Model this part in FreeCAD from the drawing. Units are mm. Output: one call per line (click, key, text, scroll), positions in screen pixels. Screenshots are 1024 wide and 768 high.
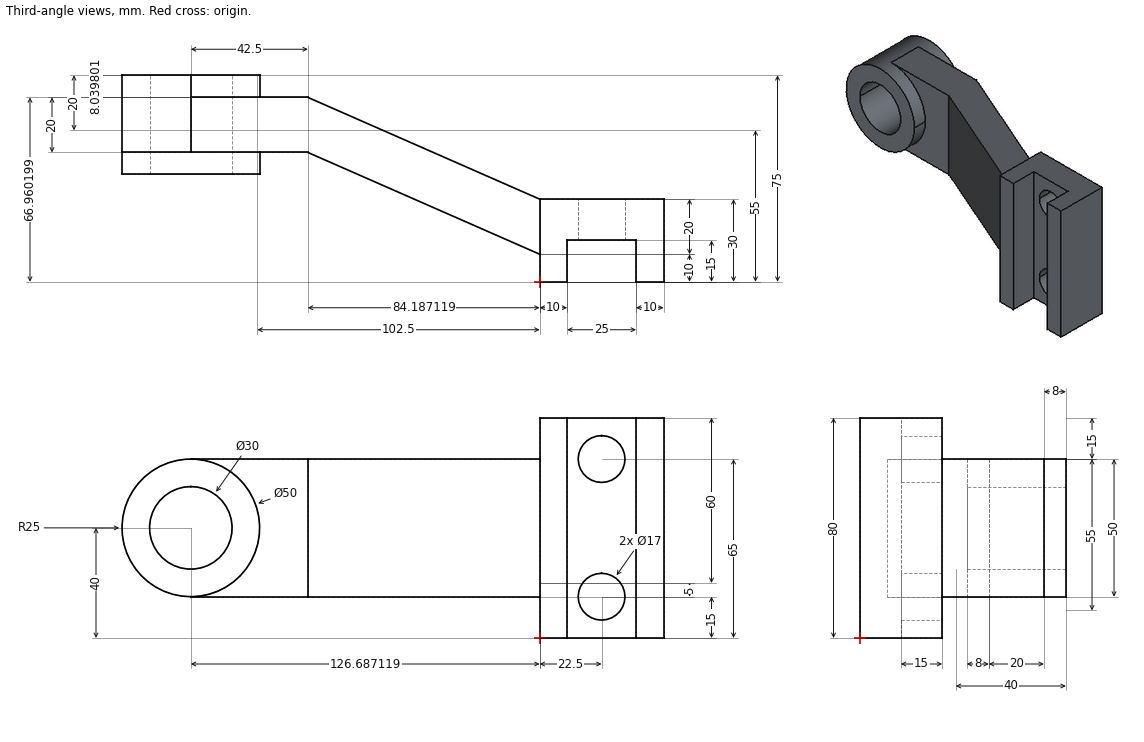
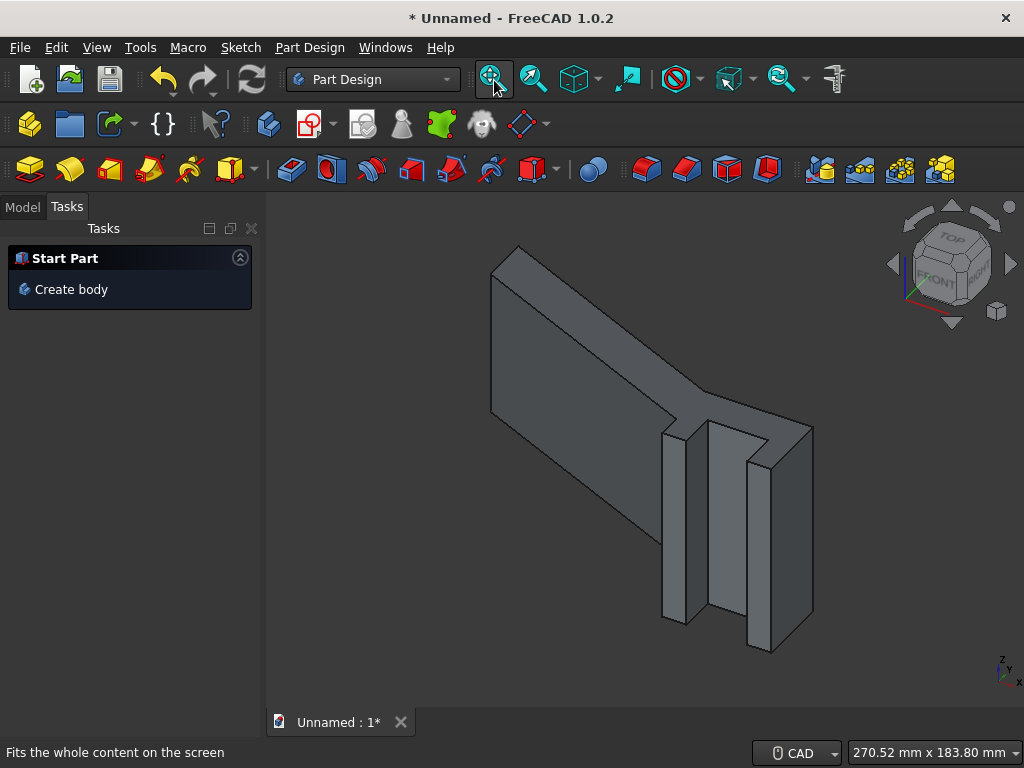
click(522, 276)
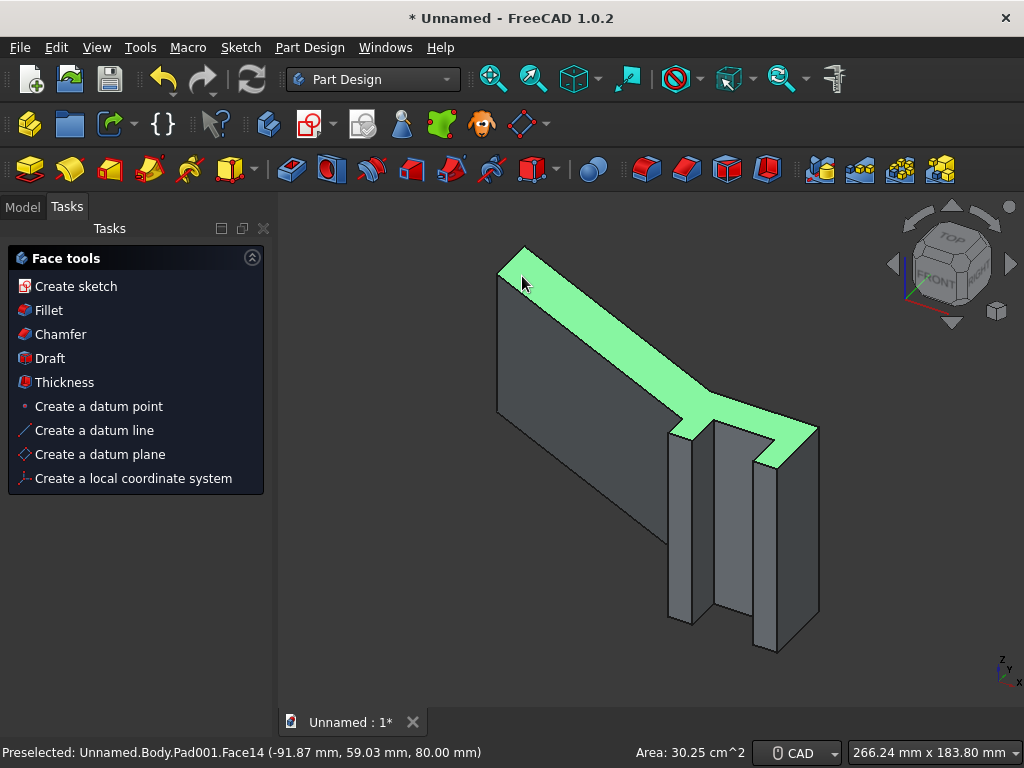
click(310, 124)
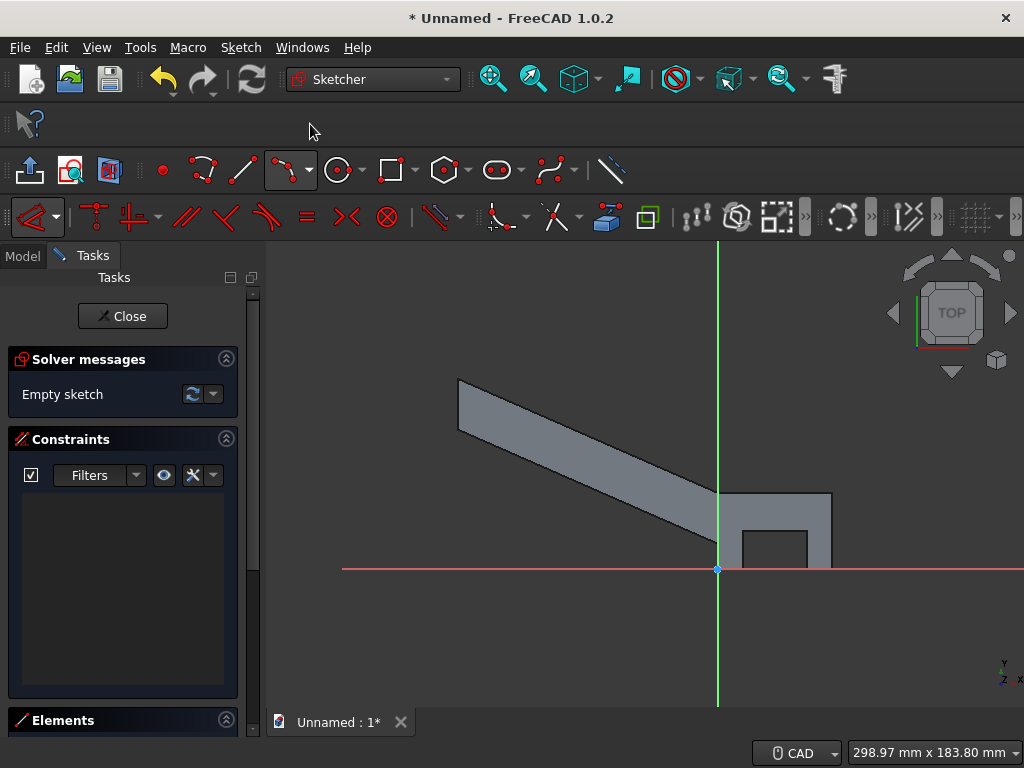
scroll(611, 474, up, 2)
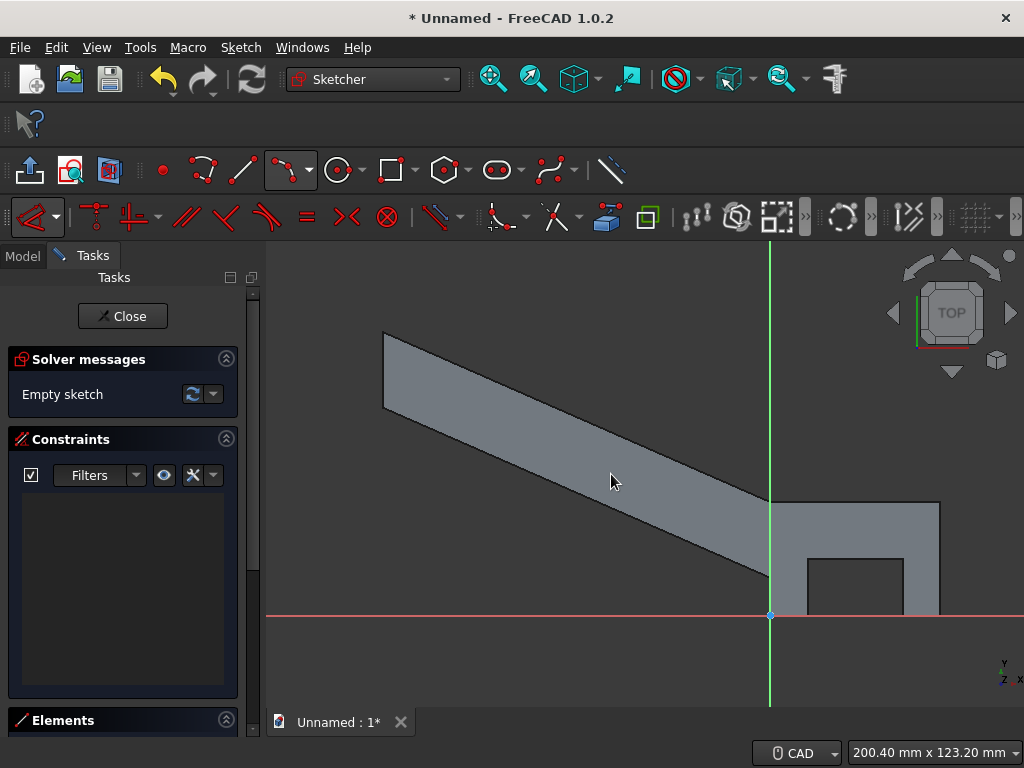
click(204, 170)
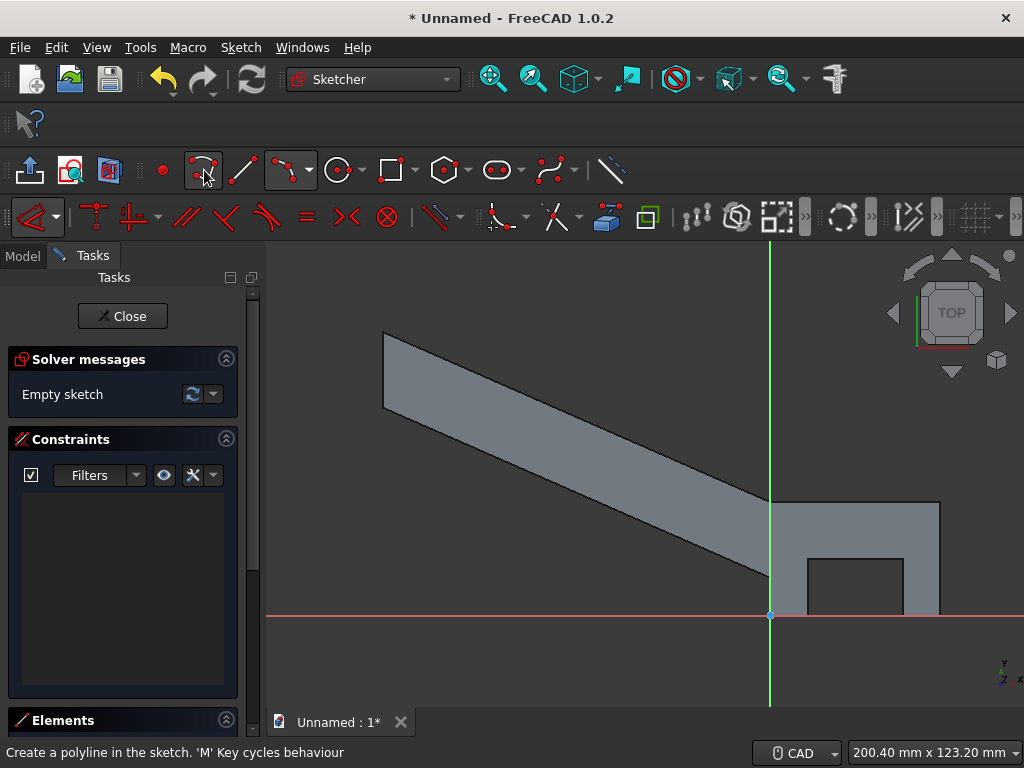
click(770, 578)
click(761, 502)
click(383, 332)
click(383, 408)
click(770, 579)
key(Escape)
key(Escape)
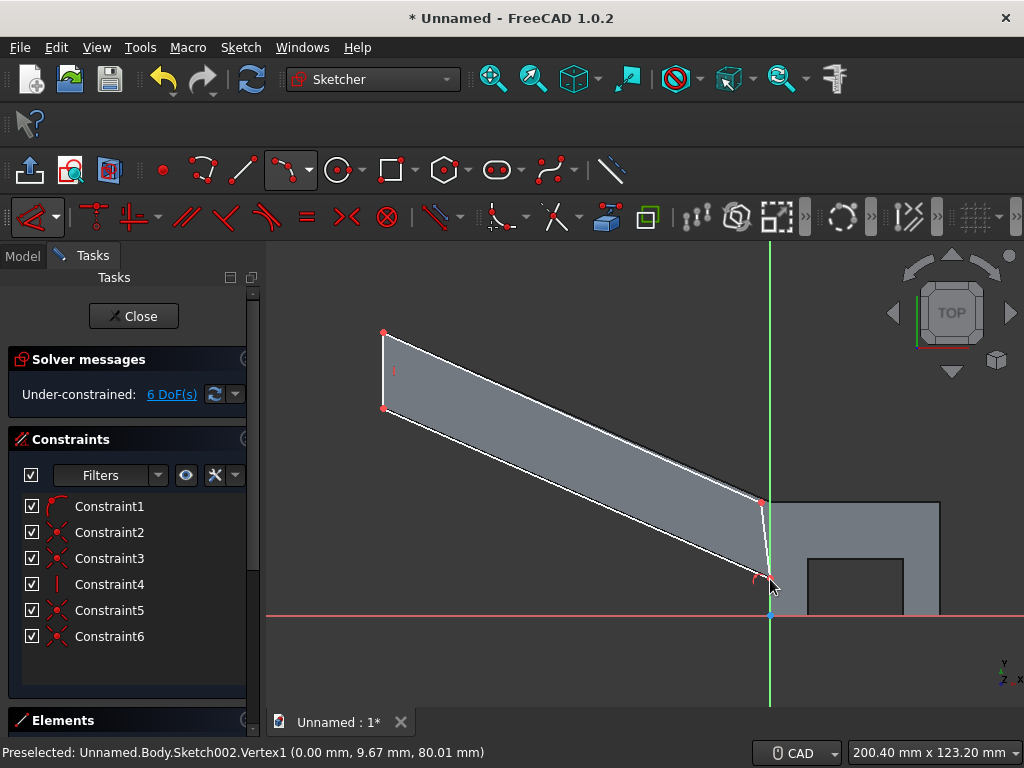
click(767, 556)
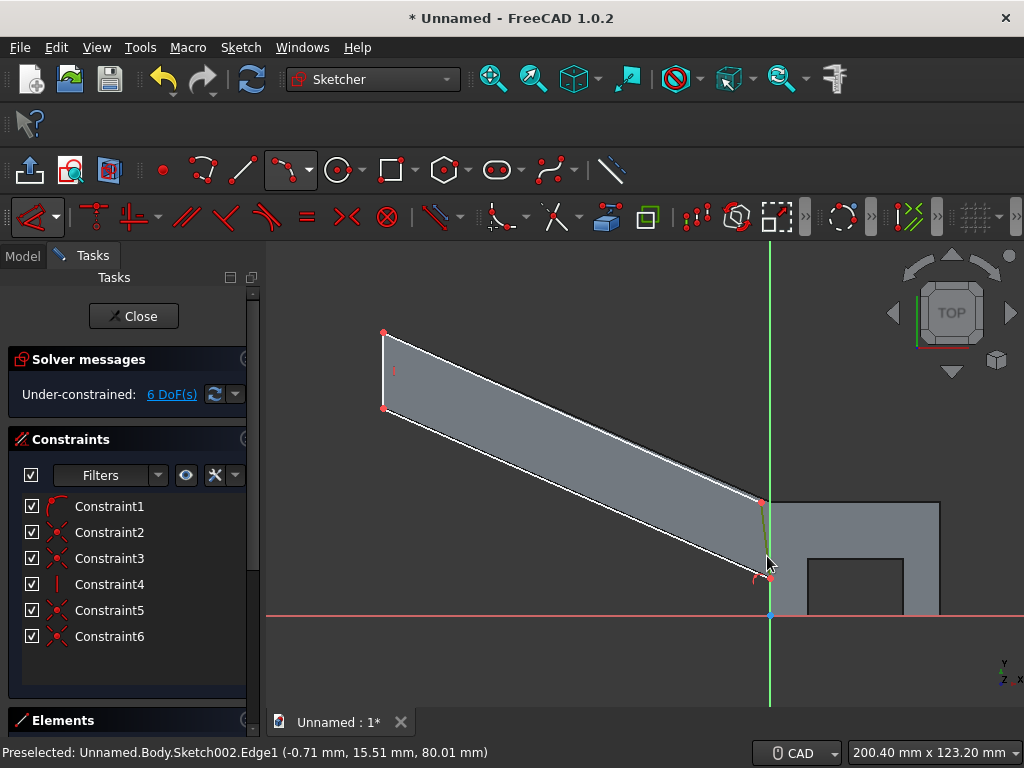
key(v)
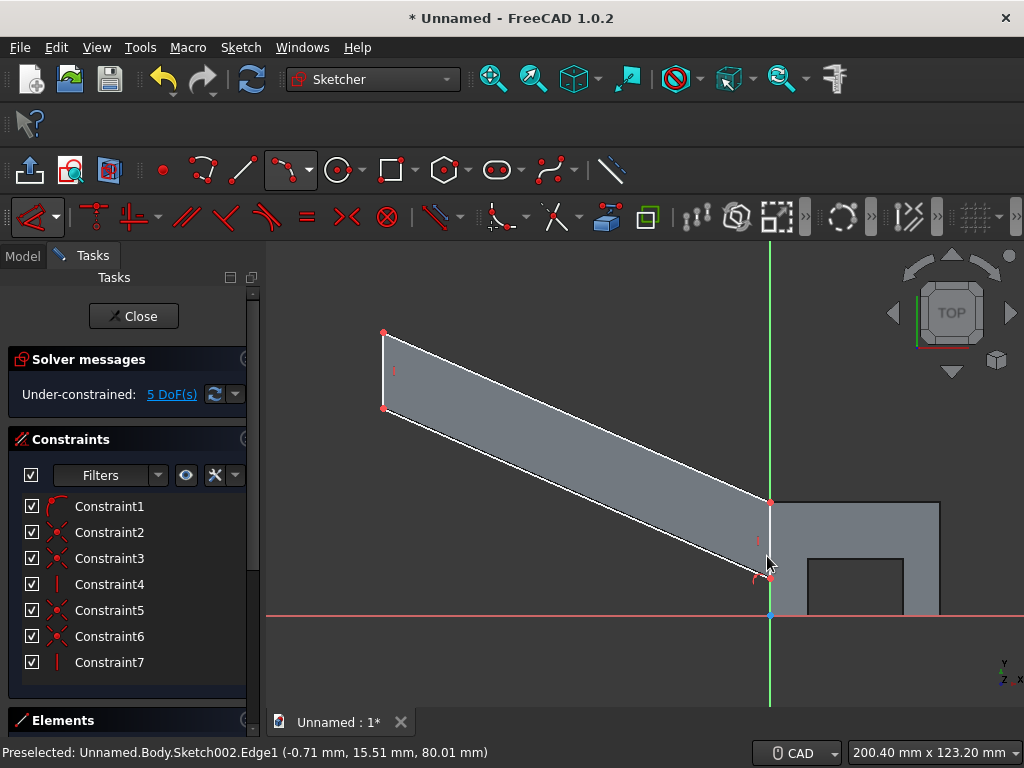
click(770, 556)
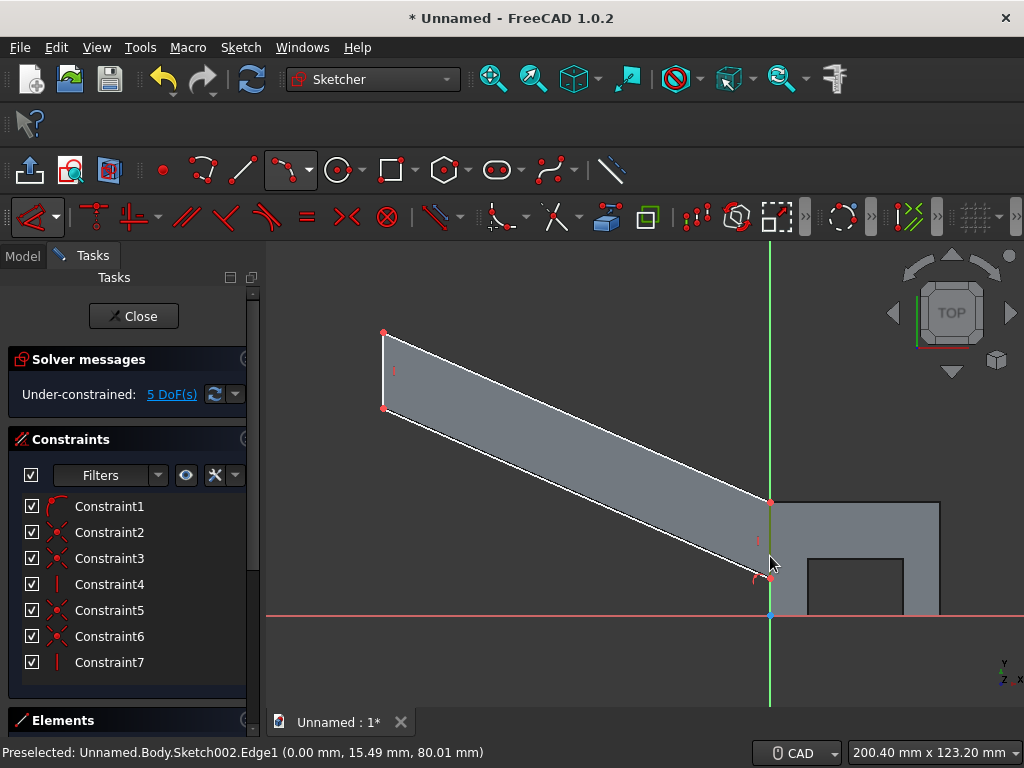
key(i)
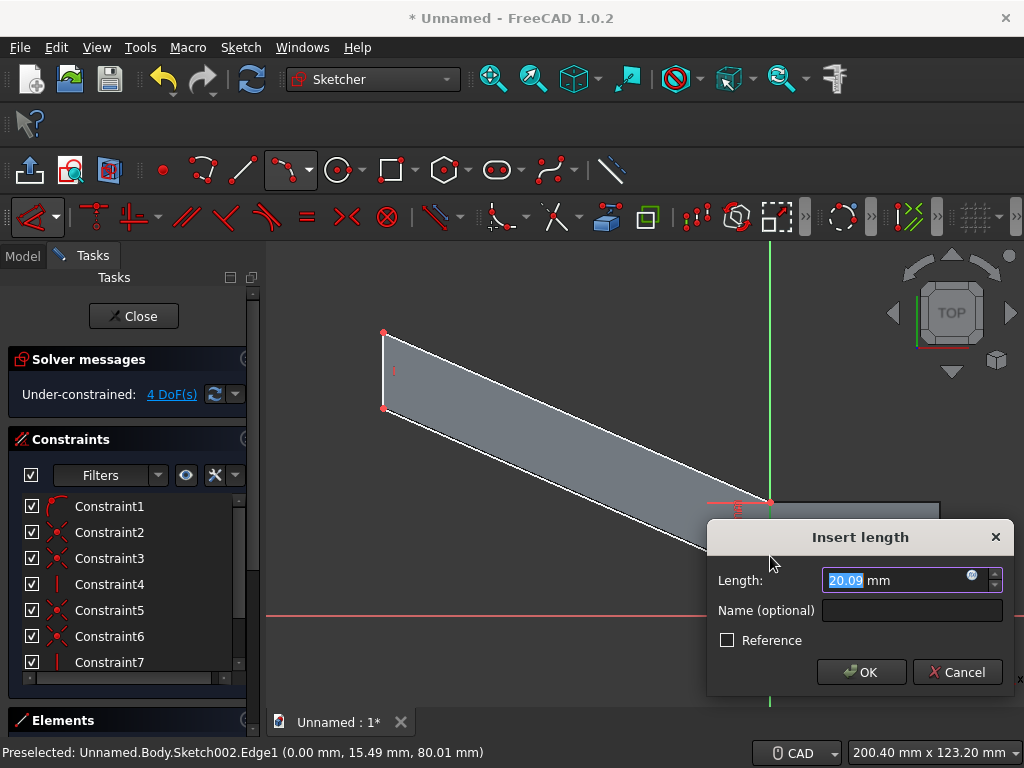
text(20)
key(Return)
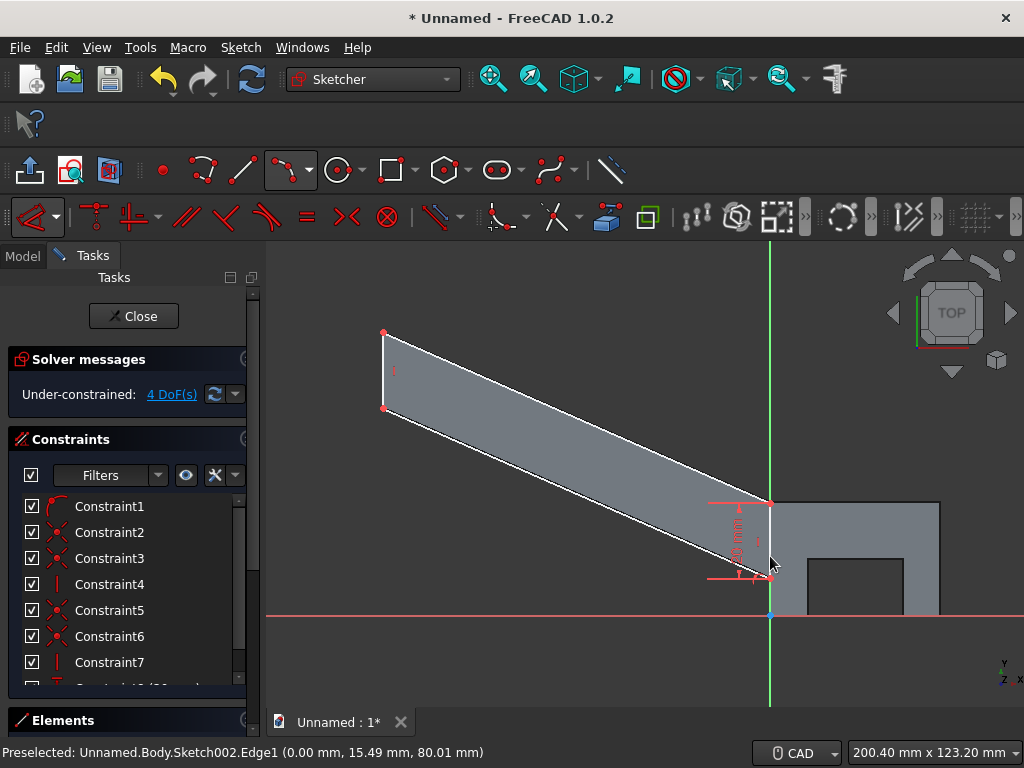
click(383, 356)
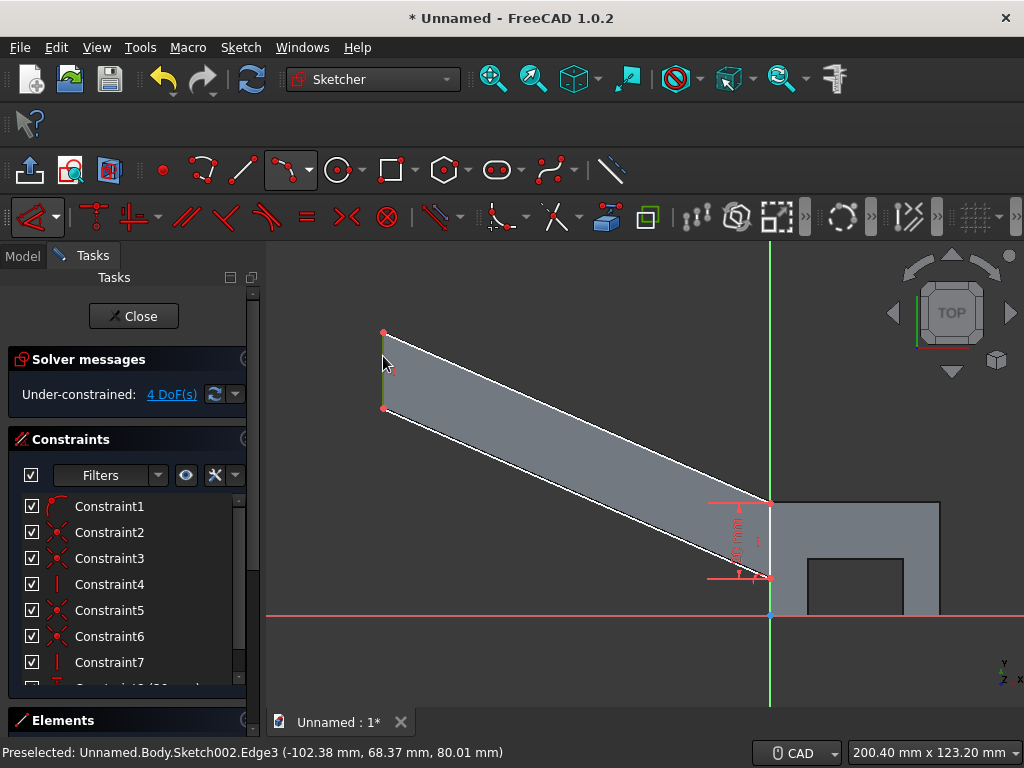
key(i)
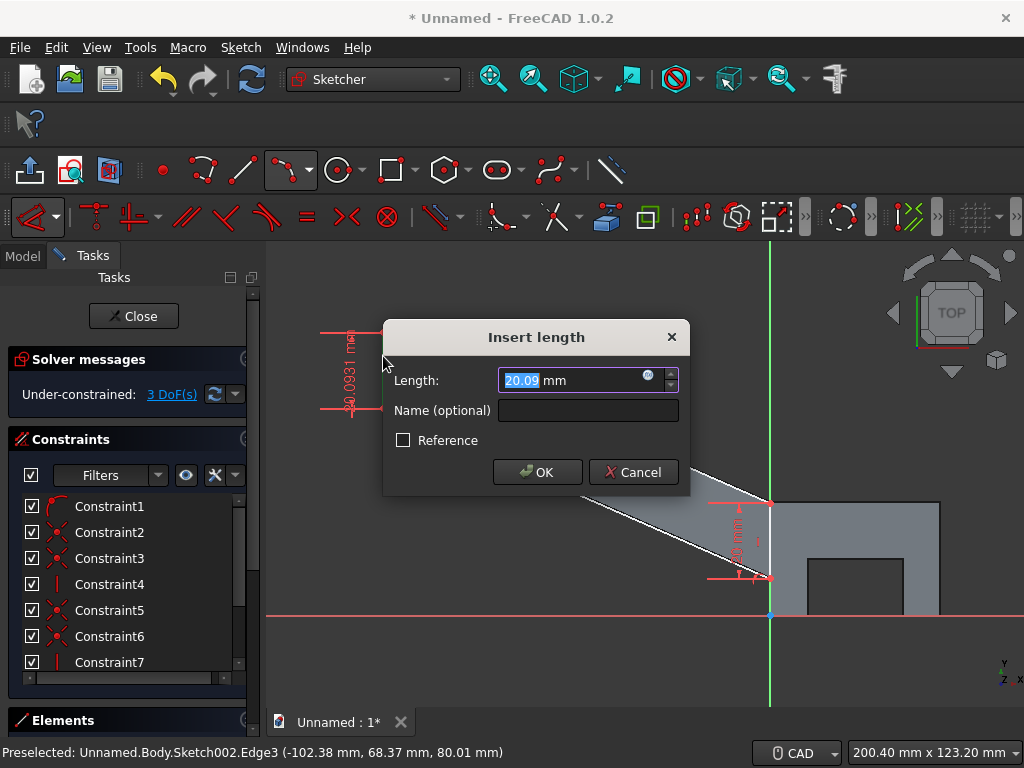
text(20)
key(Return)